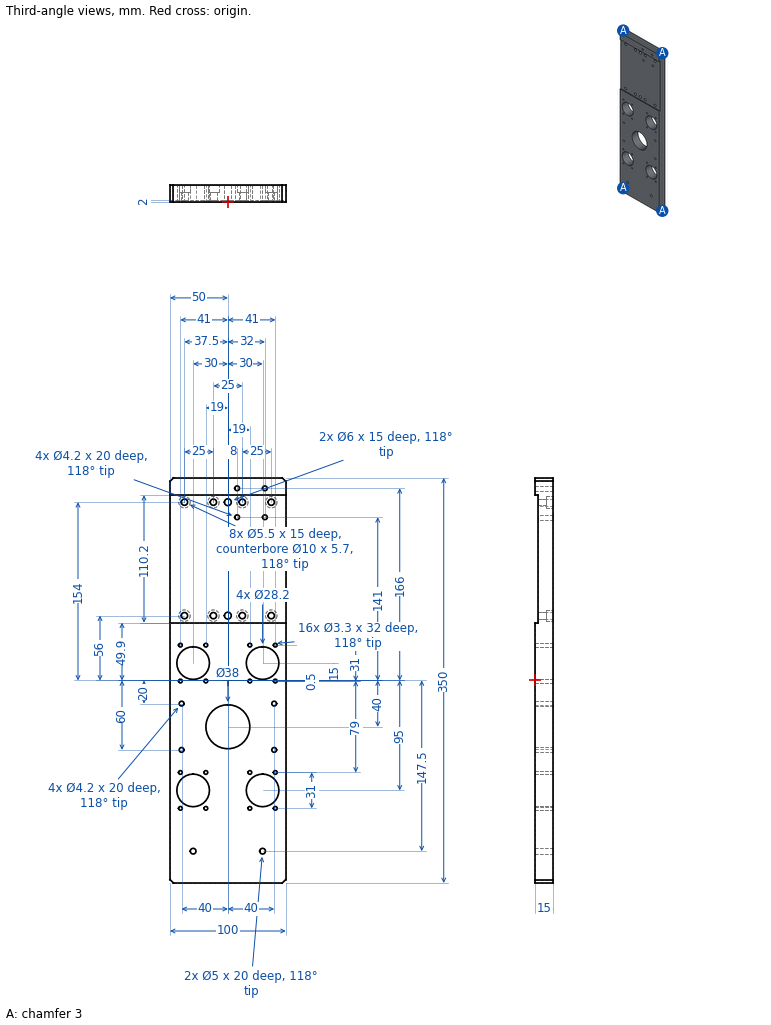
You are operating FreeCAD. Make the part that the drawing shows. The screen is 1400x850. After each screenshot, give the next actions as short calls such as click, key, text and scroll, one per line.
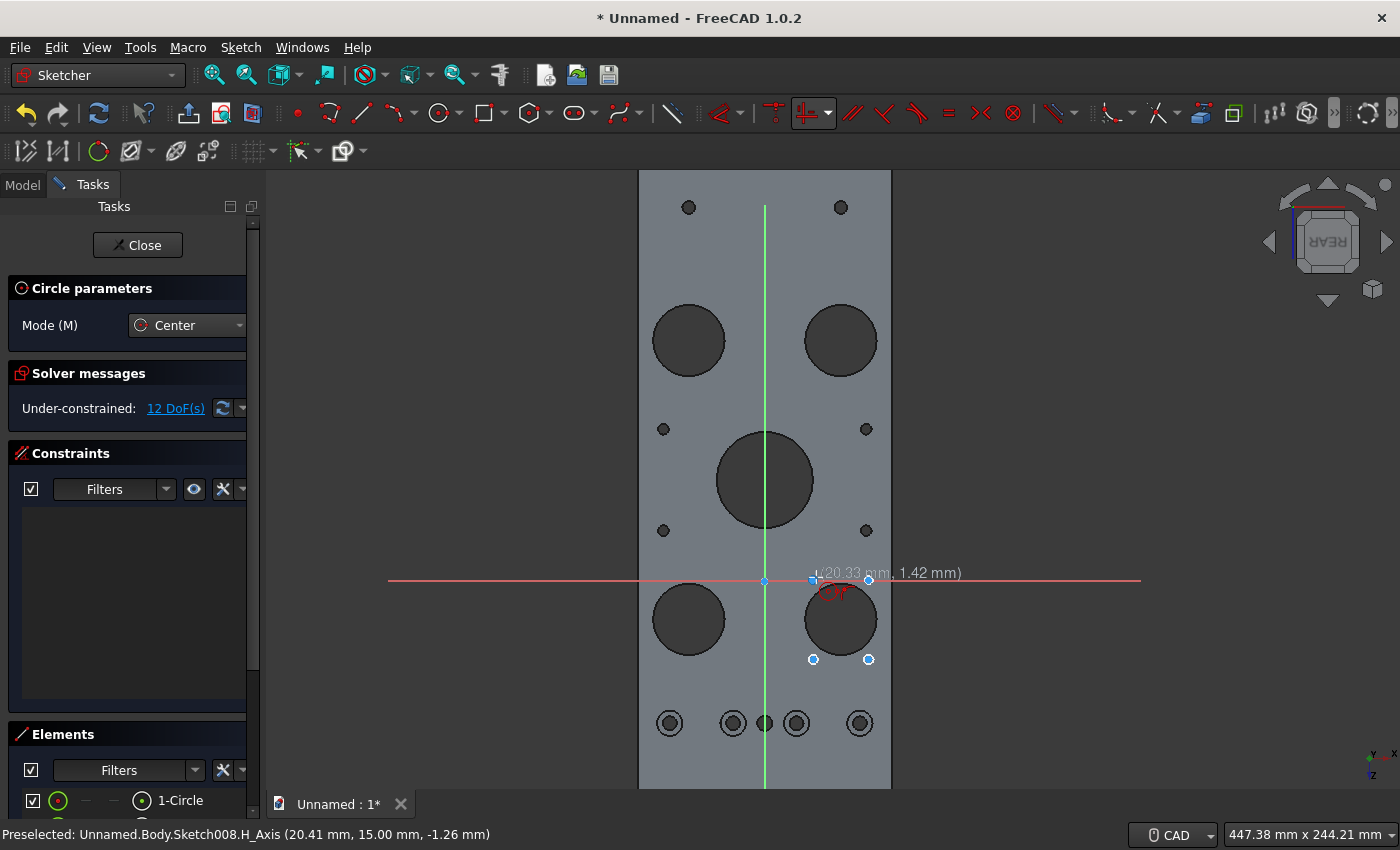
scroll(717, 659, up, 9)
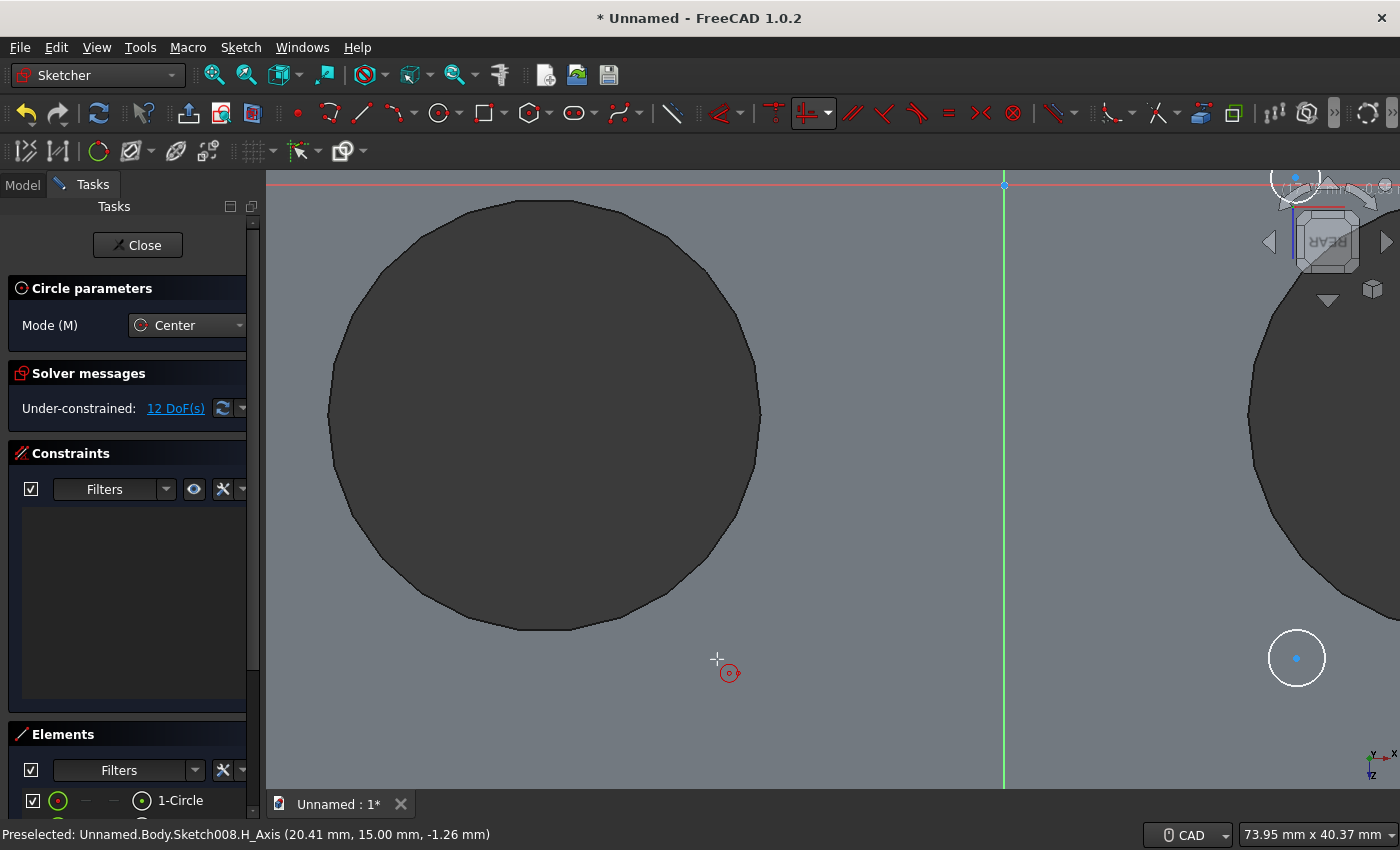
scroll(717, 659, down, 9)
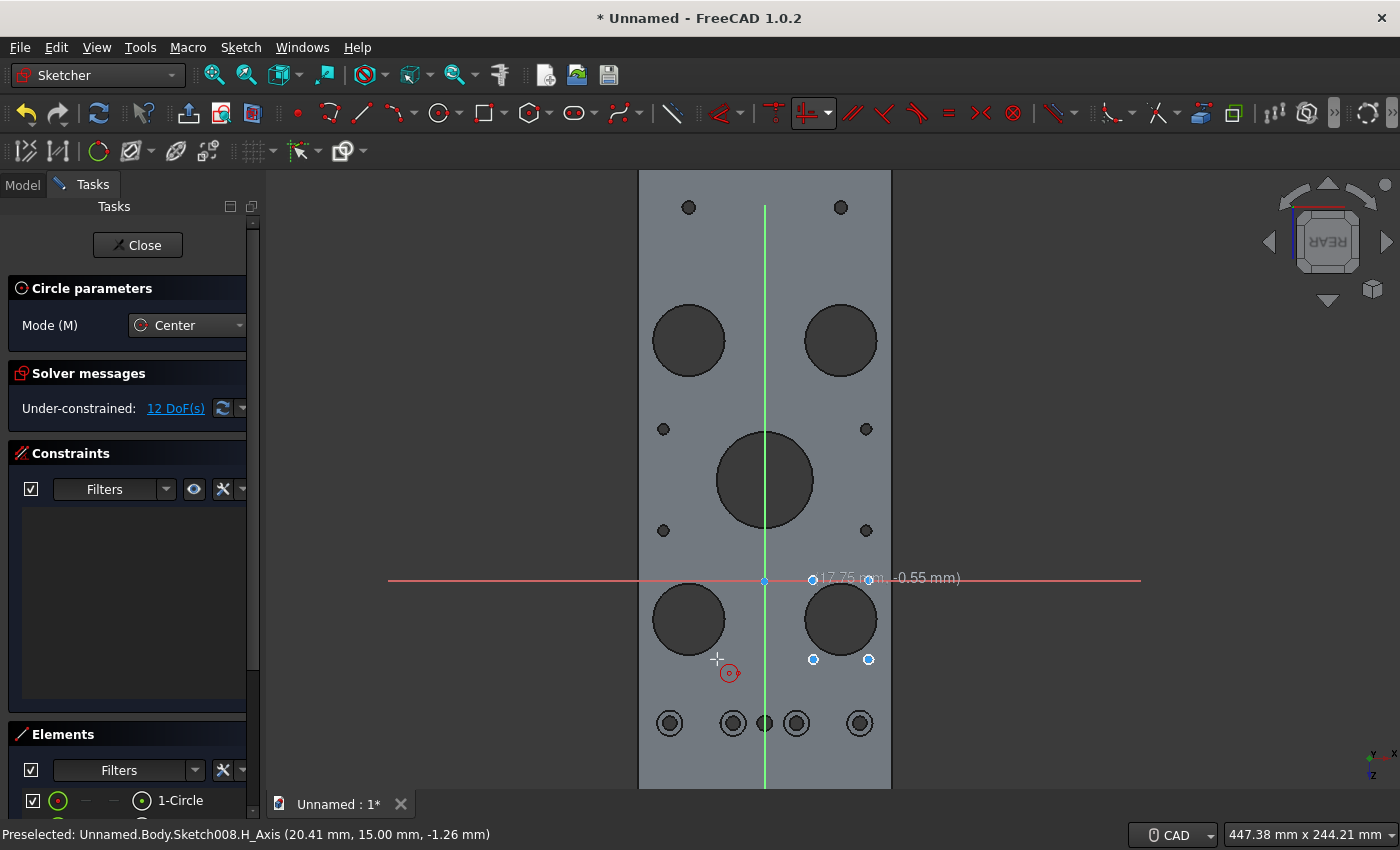
click(717, 659)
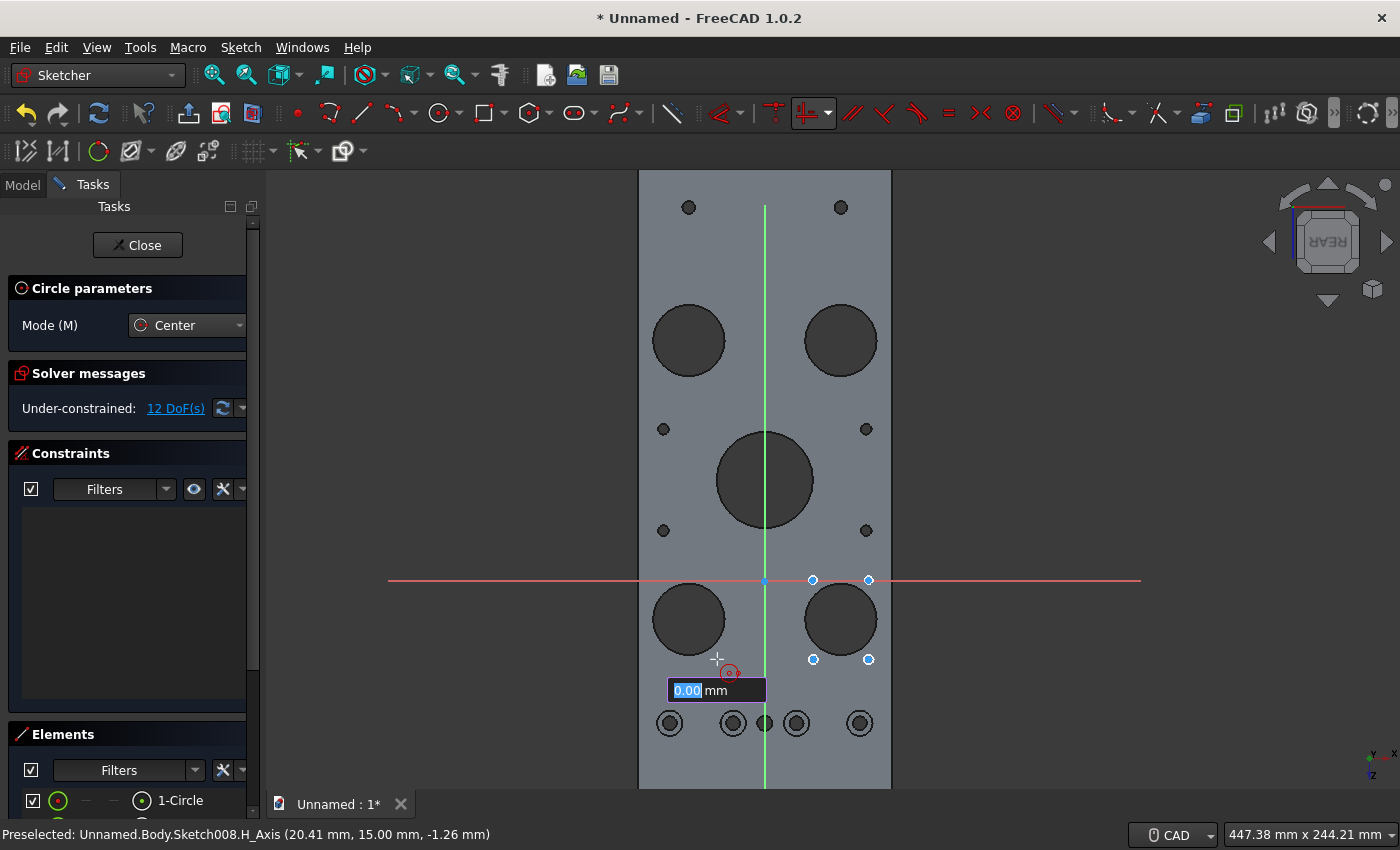
scroll(720, 656, up, 7)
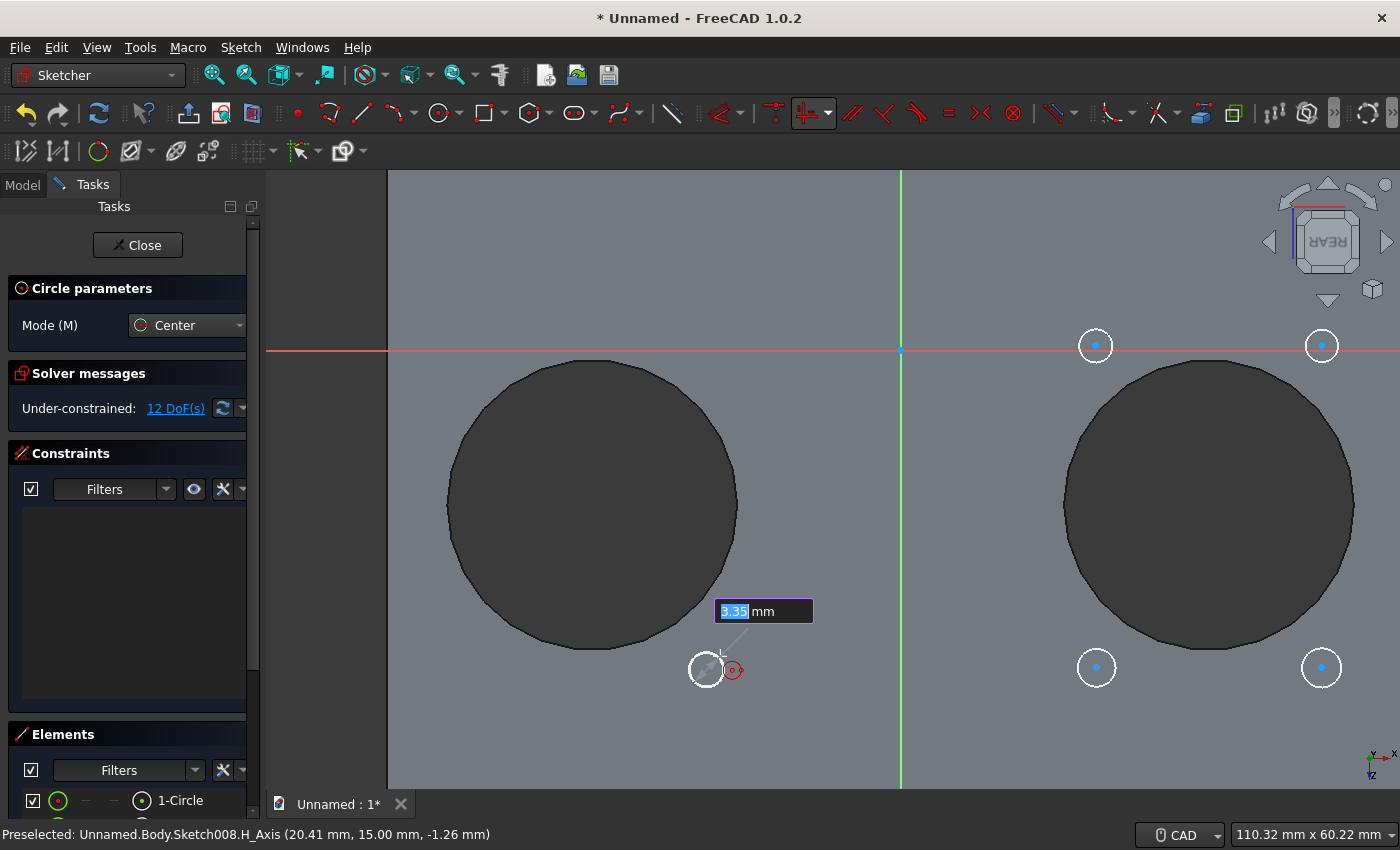
click(717, 652)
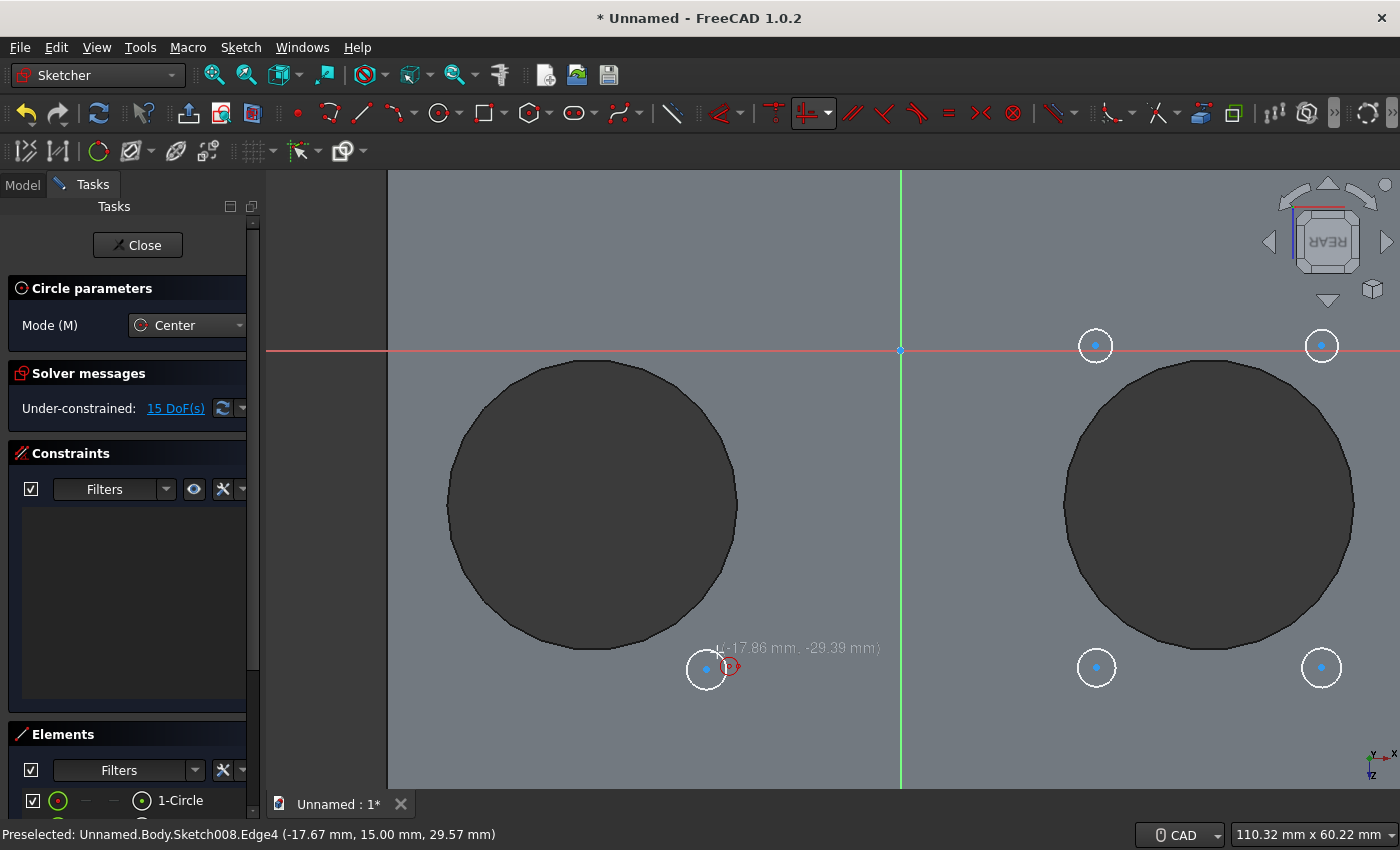
scroll(479, 664, up, 2)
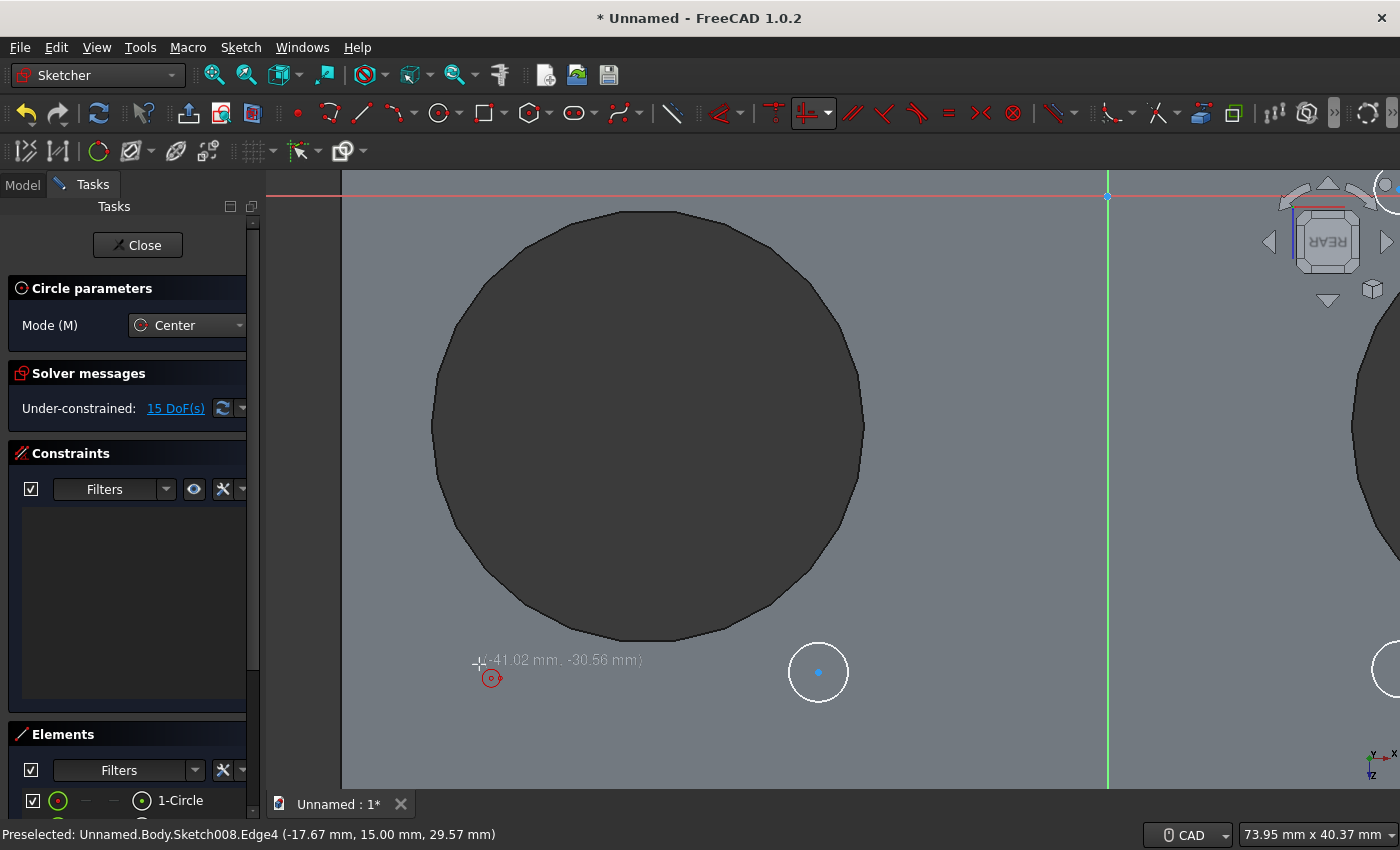
scroll(696, 657, down, 9)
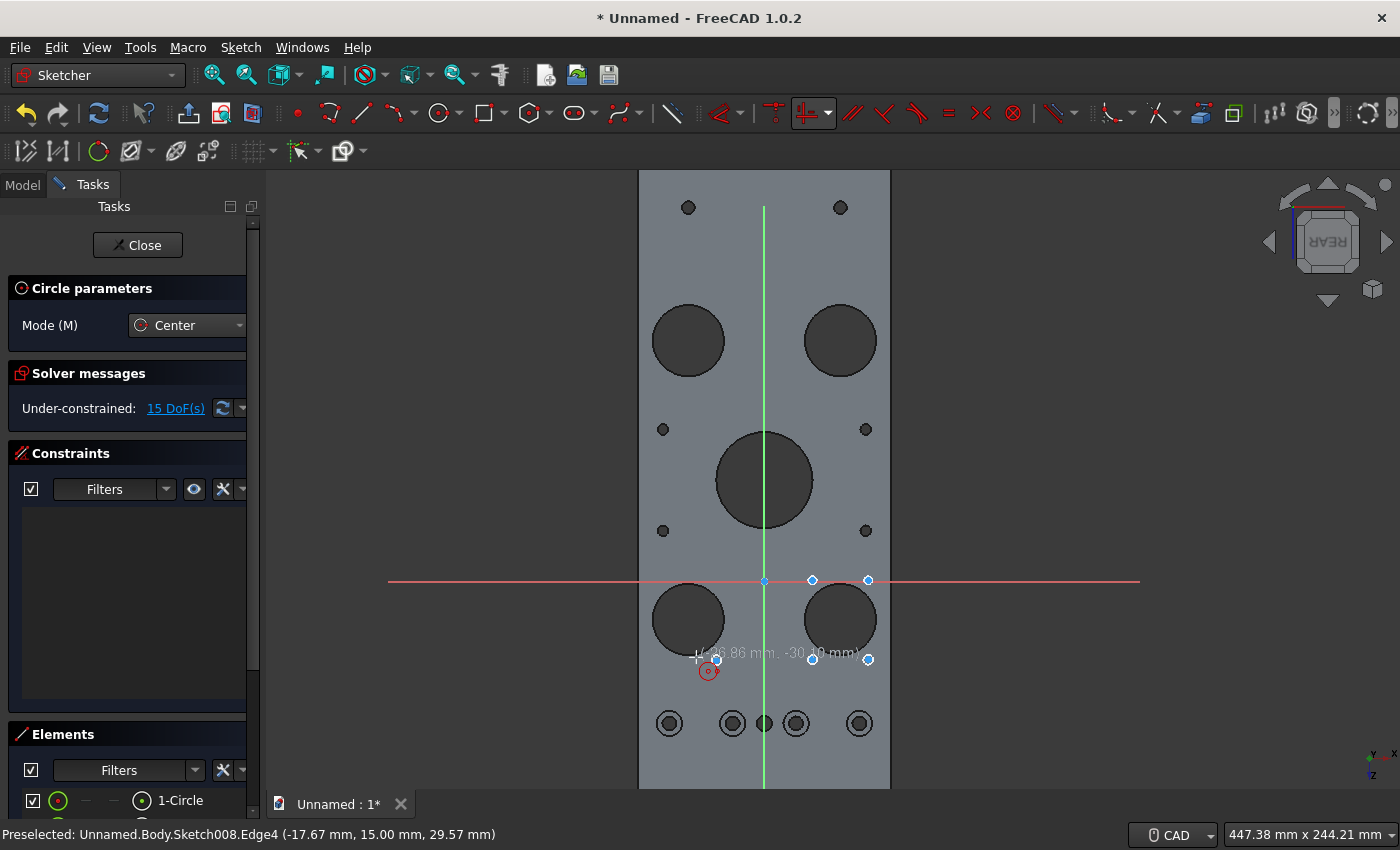
click(660, 659)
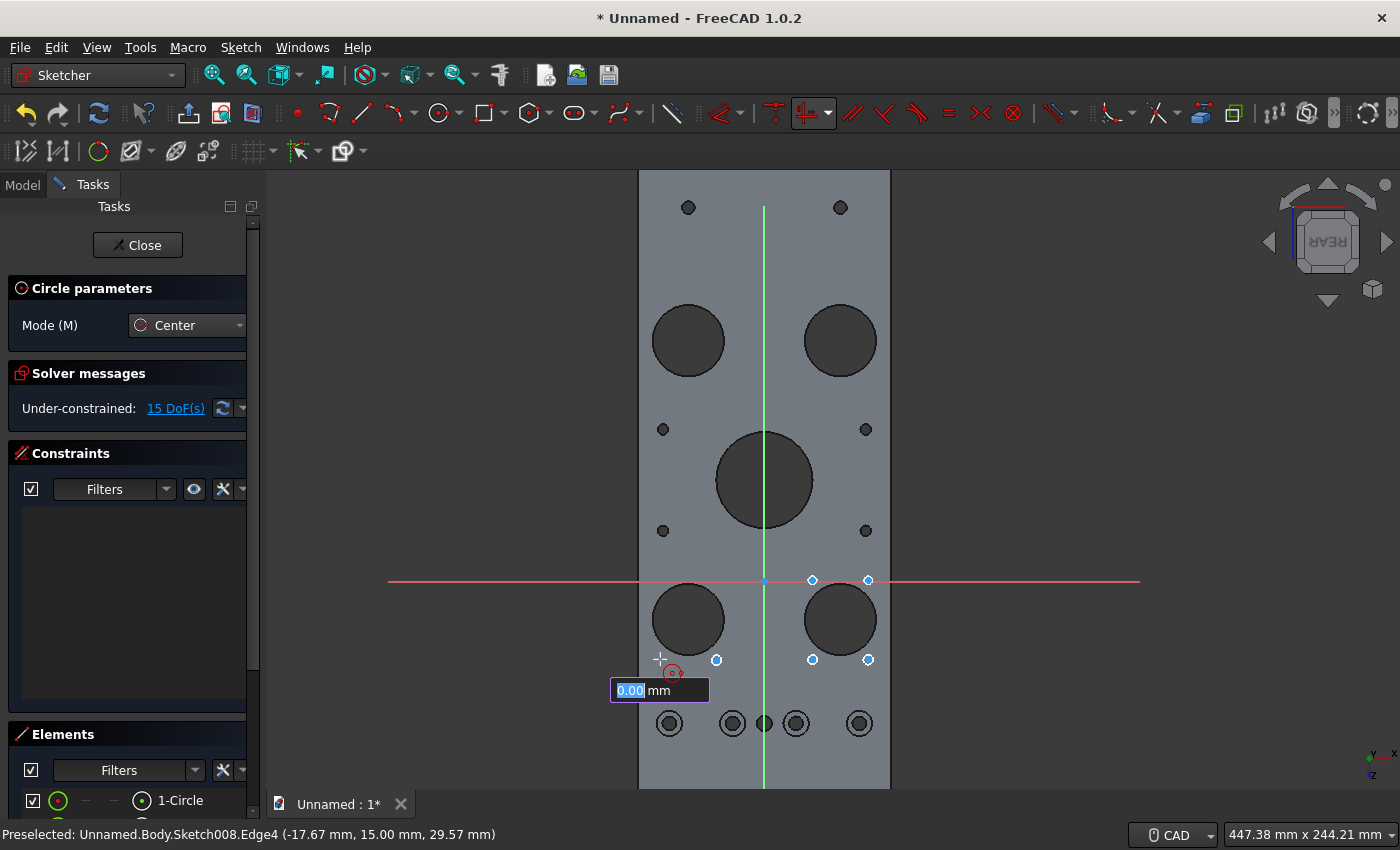
scroll(663, 656, up, 7)